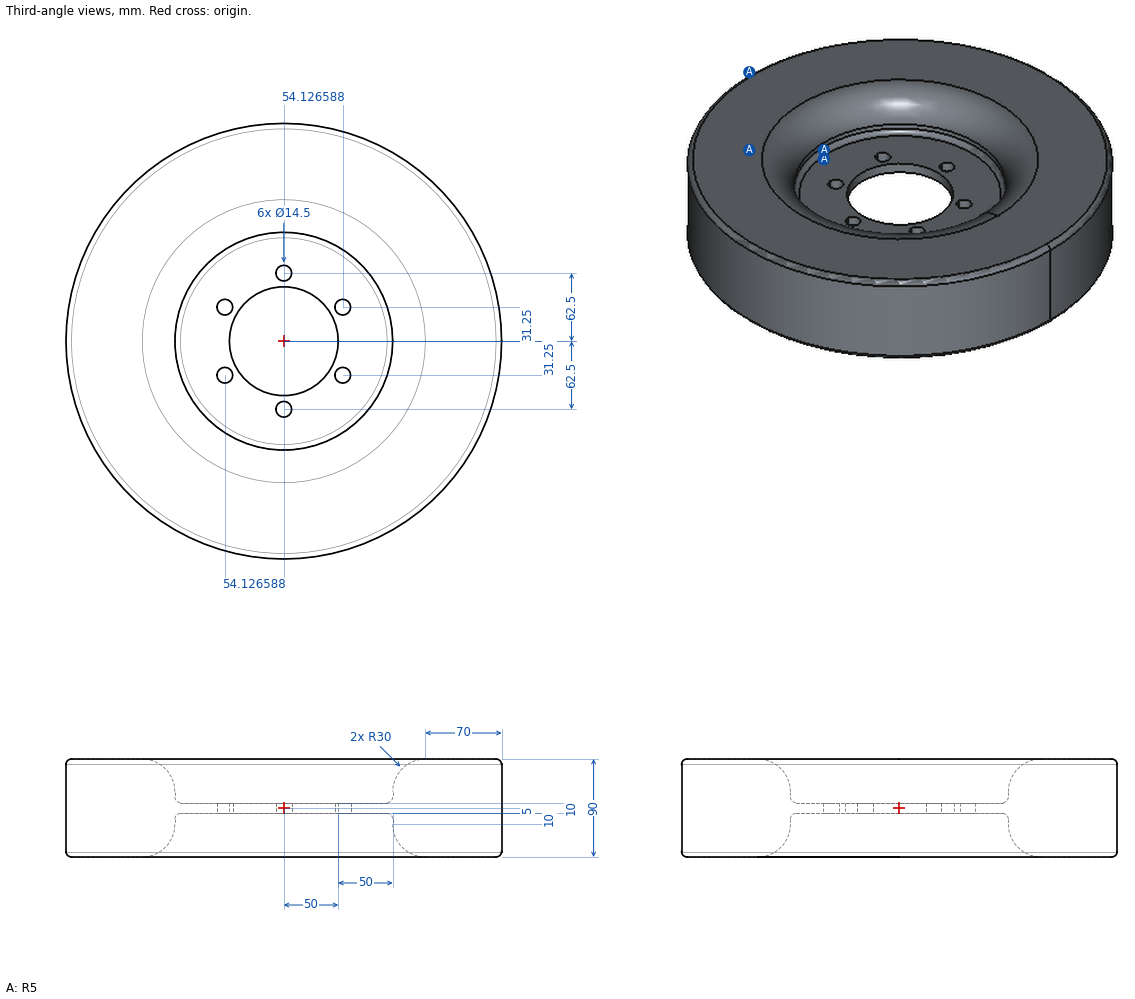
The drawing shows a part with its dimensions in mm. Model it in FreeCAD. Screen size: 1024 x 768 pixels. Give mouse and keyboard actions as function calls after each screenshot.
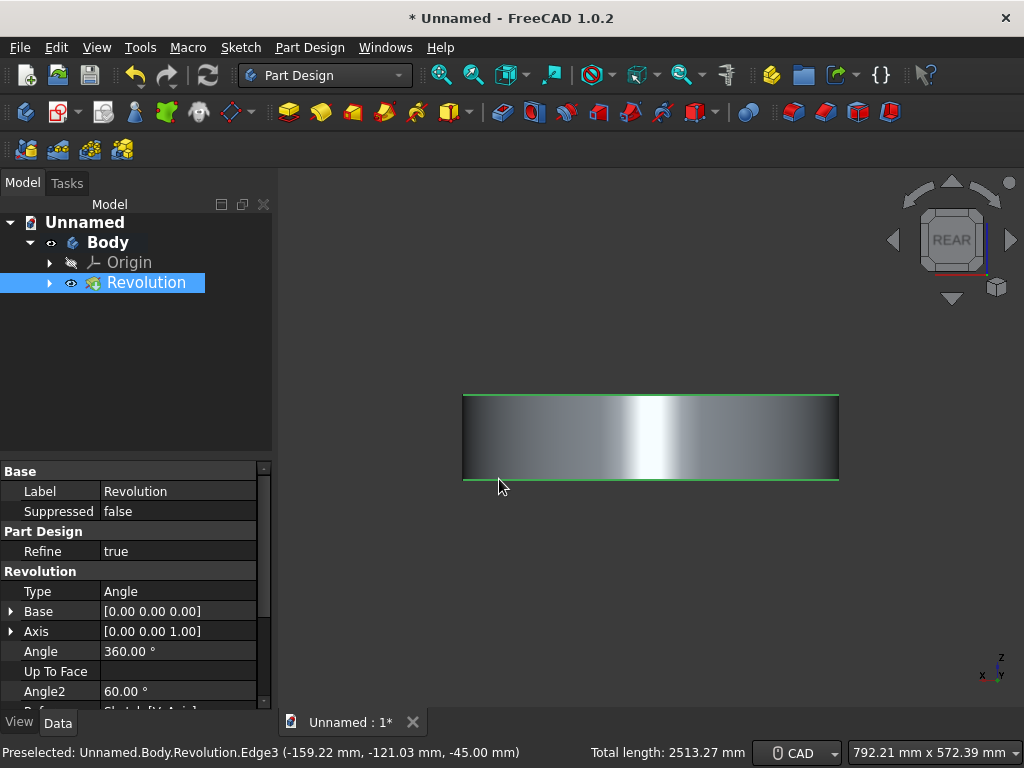
key(6)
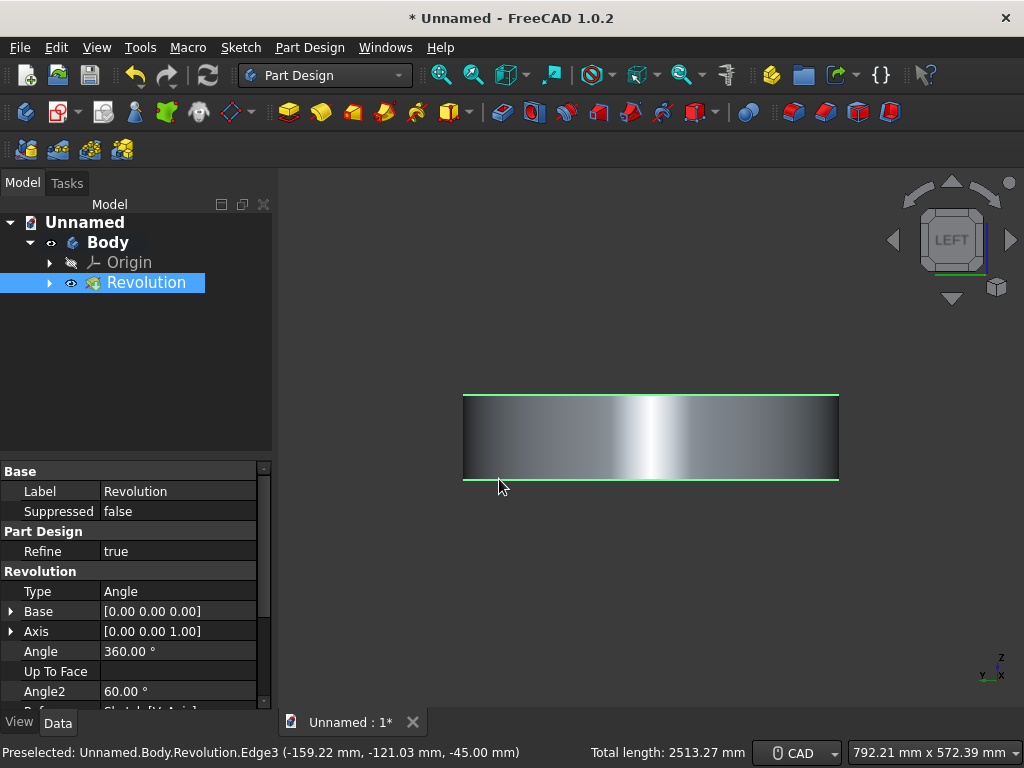
key(v)
key(3)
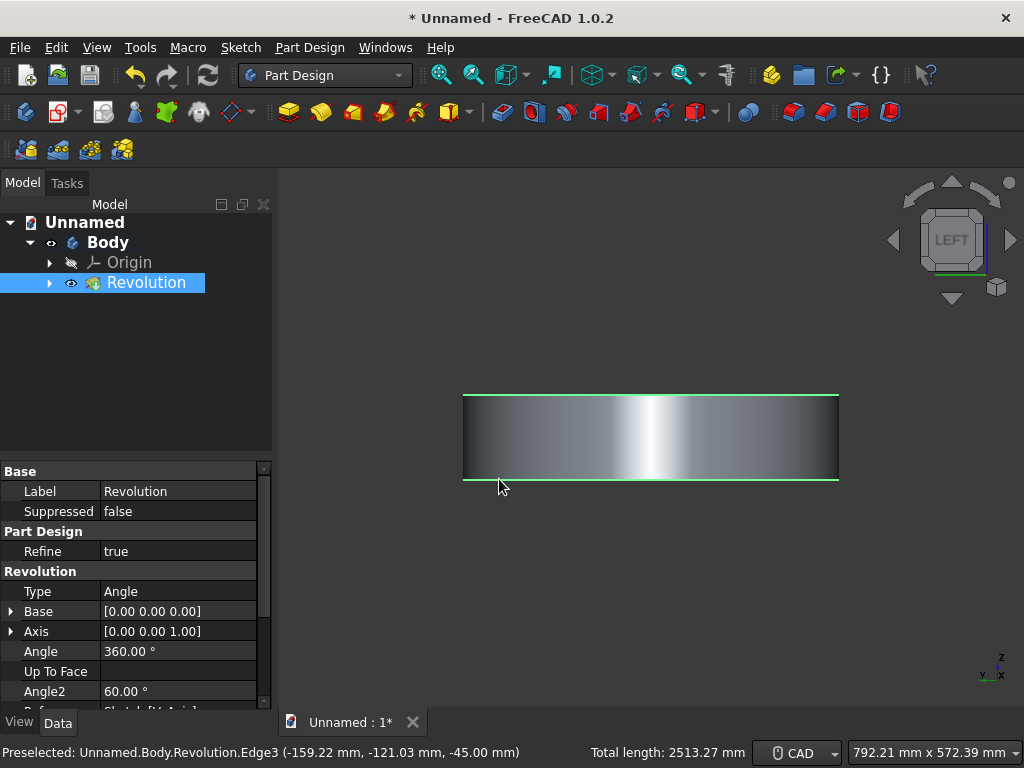
key(0)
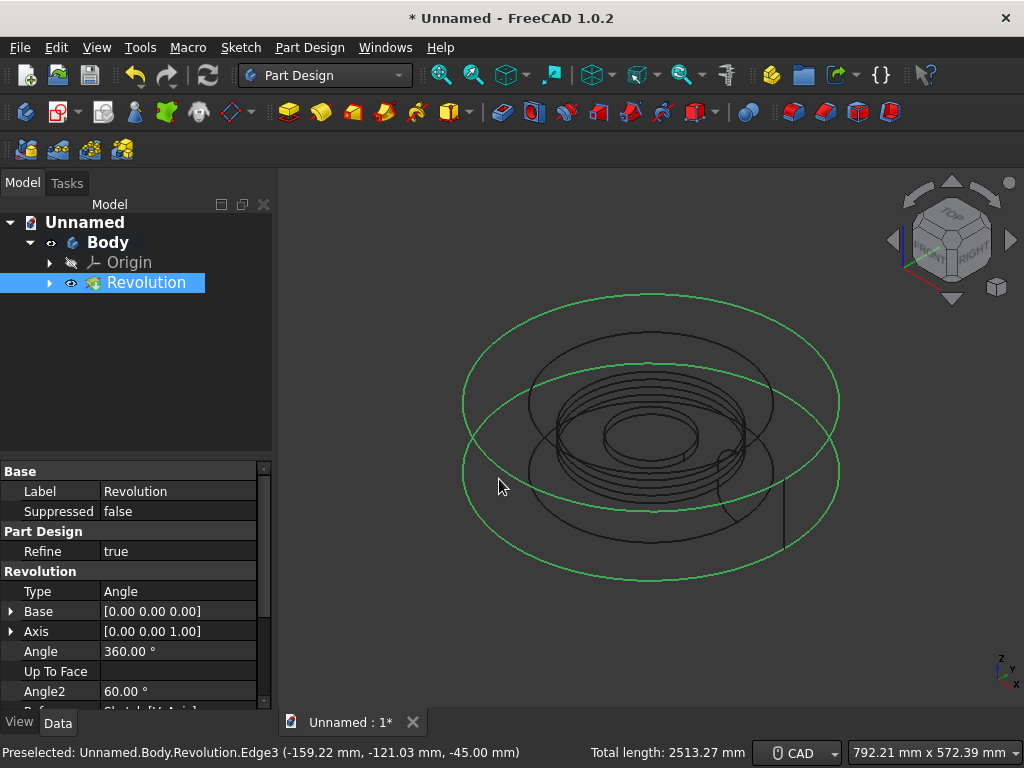
click(636, 387, ctrl)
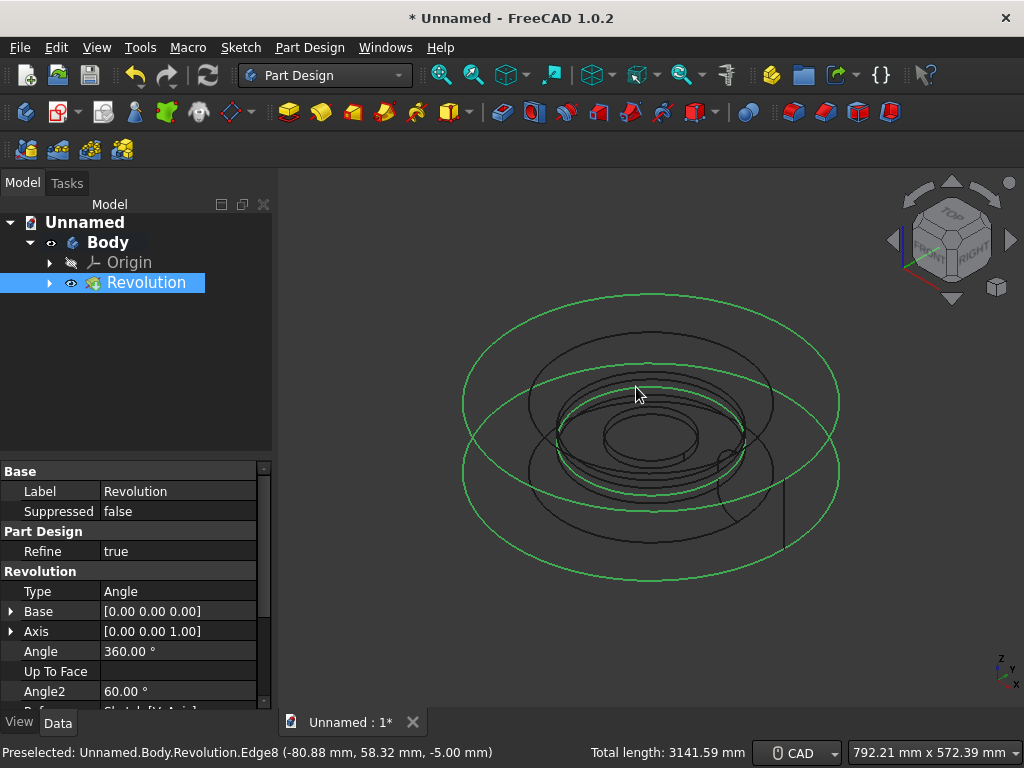
click(636, 379, ctrl)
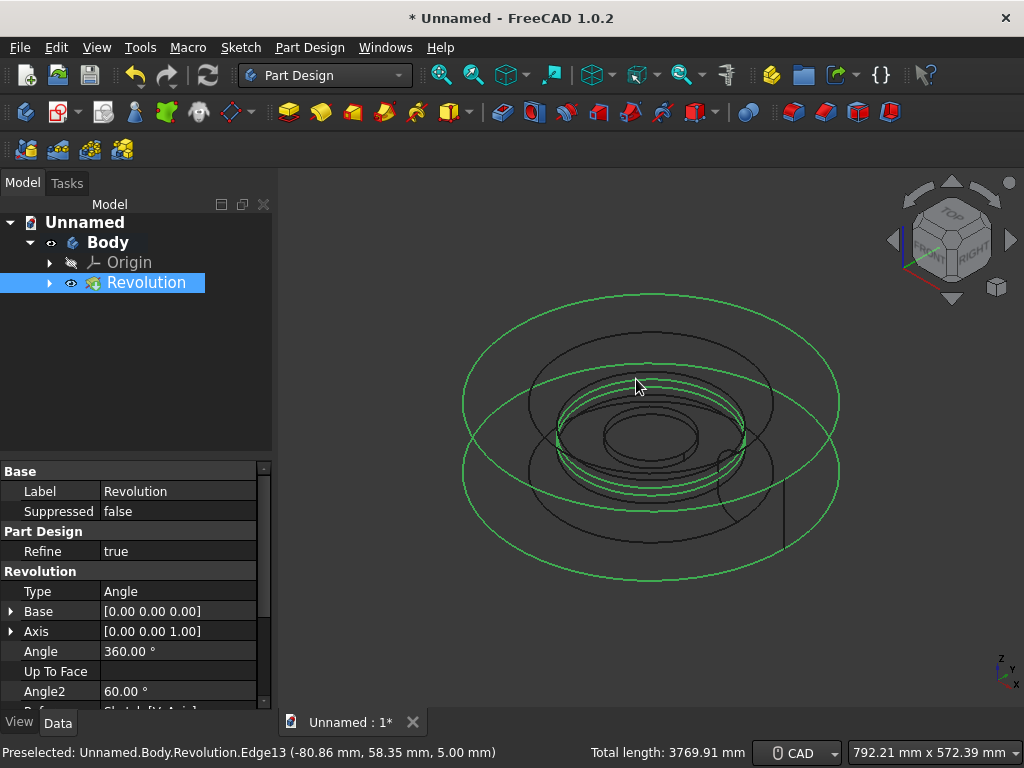
key(v)
key(1)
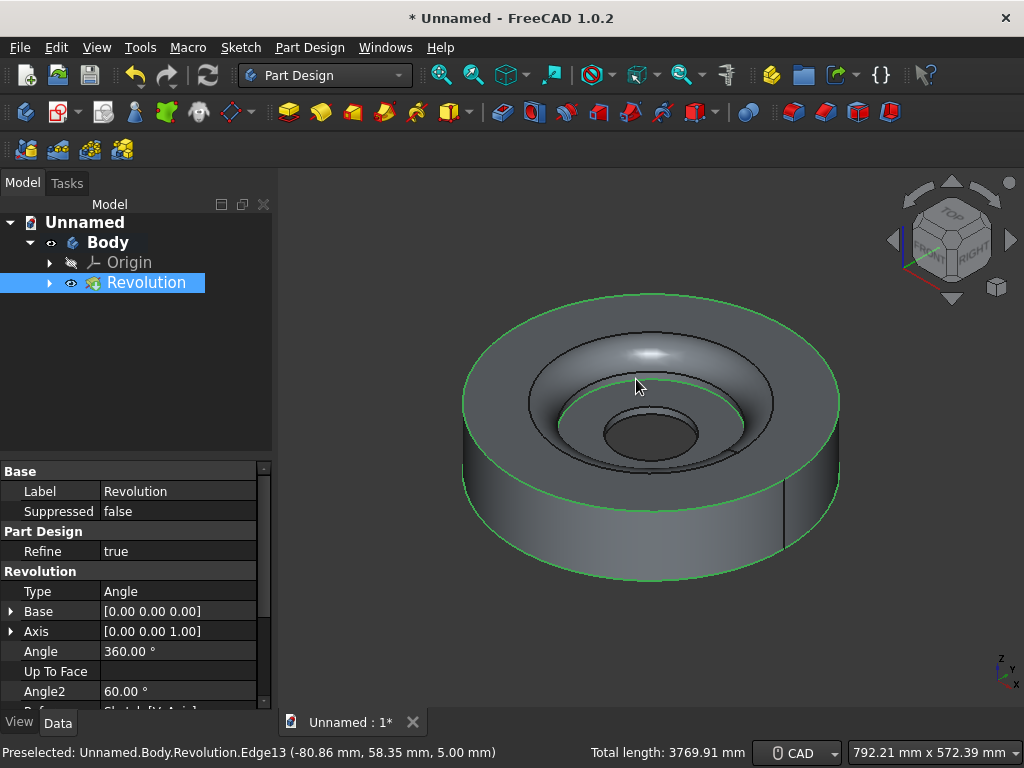
click(794, 112)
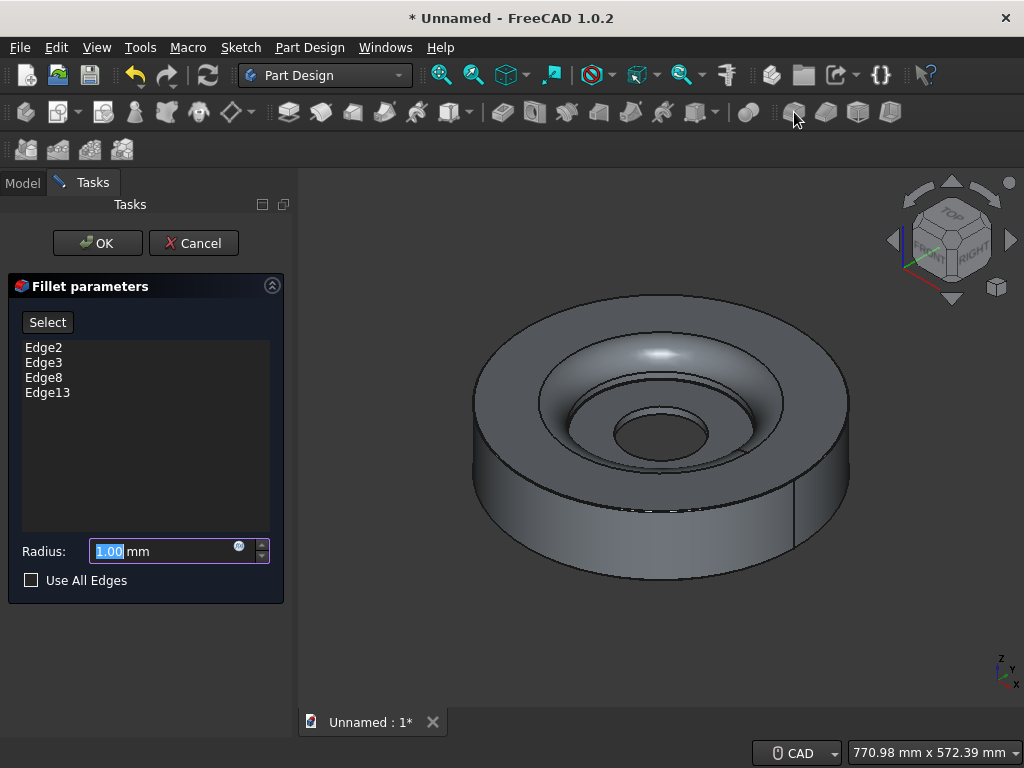
text(5)
key(Tab)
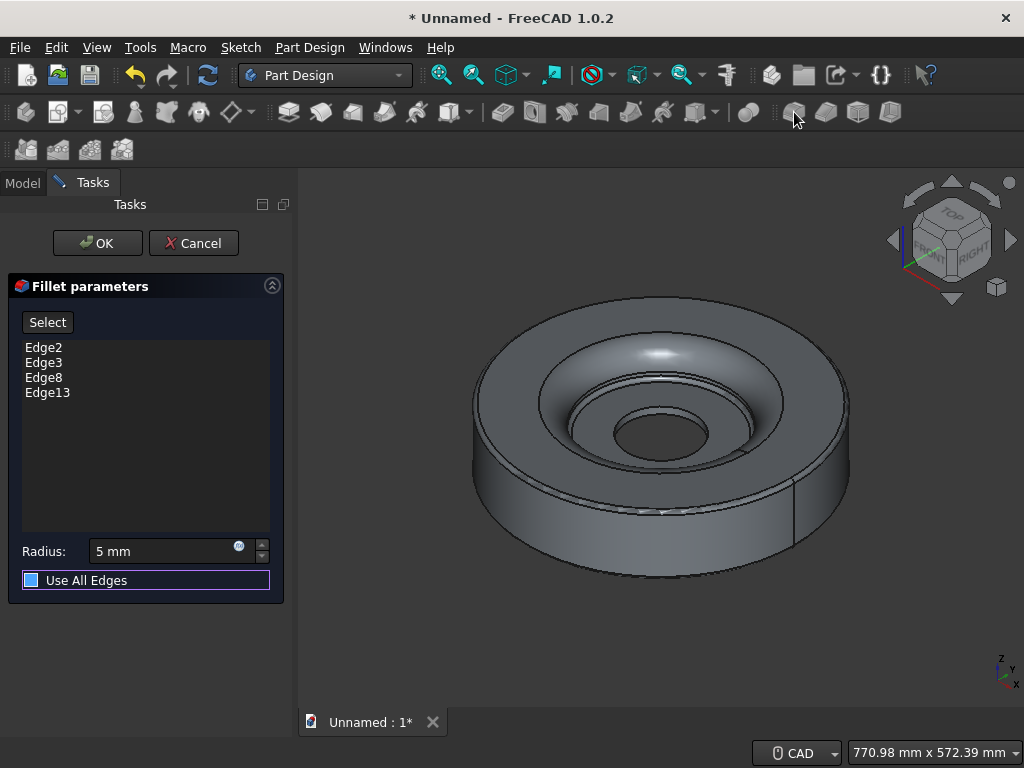
click(98, 243)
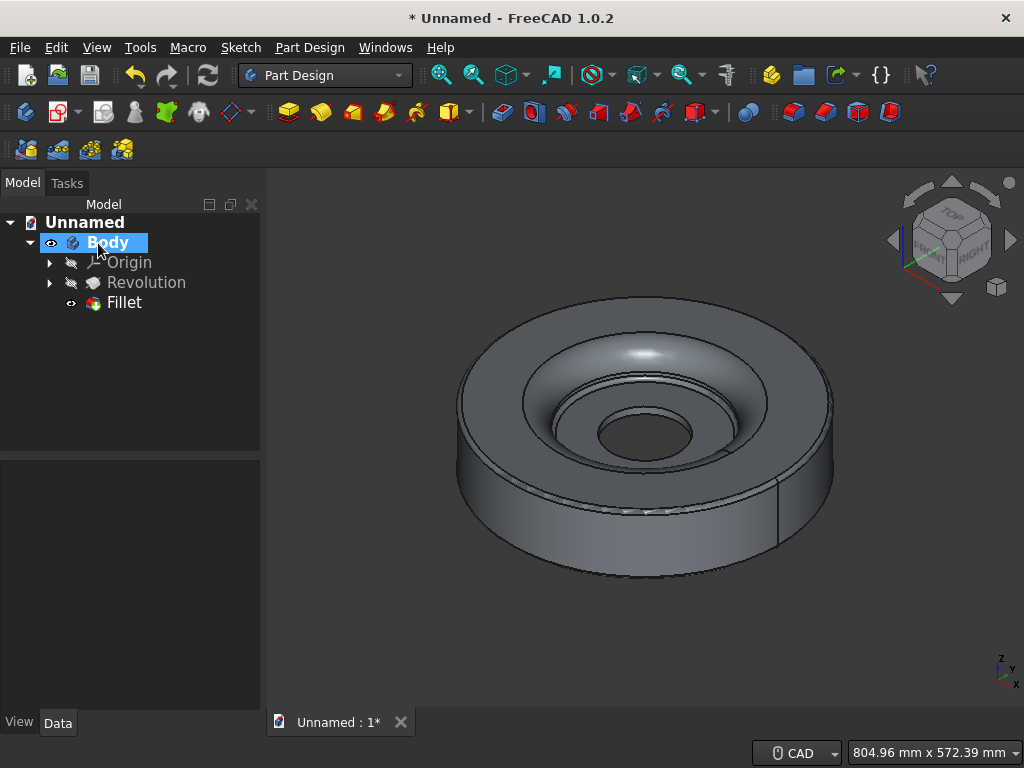
click(645, 391)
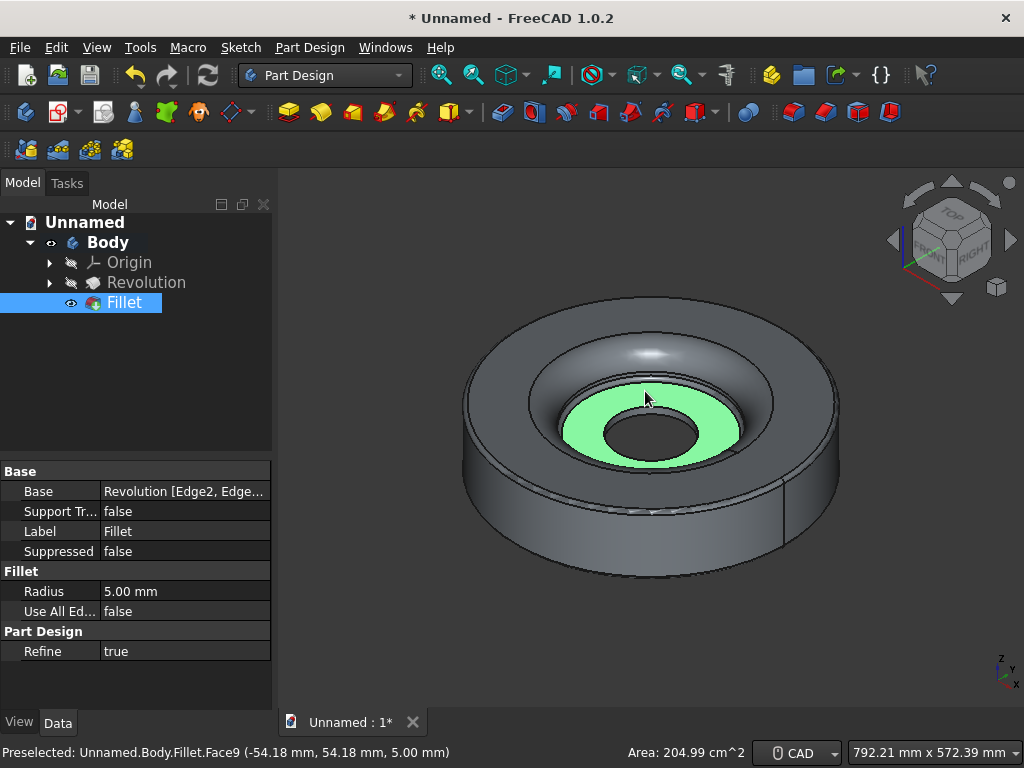
click(58, 112)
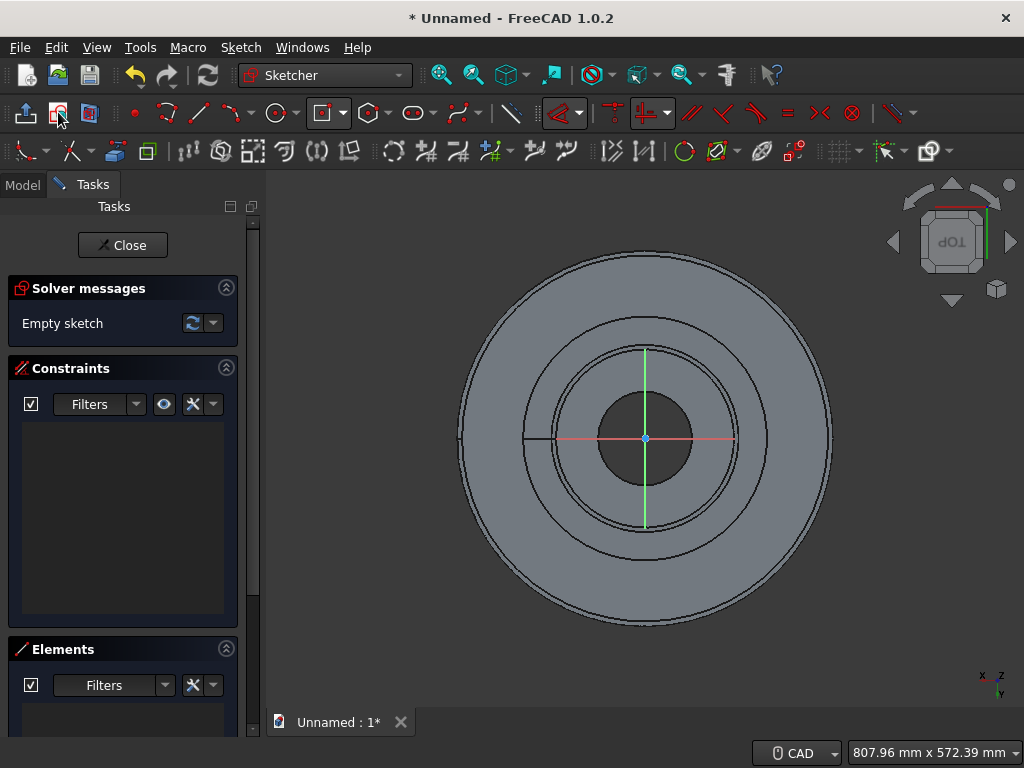
scroll(685, 439, up, 5)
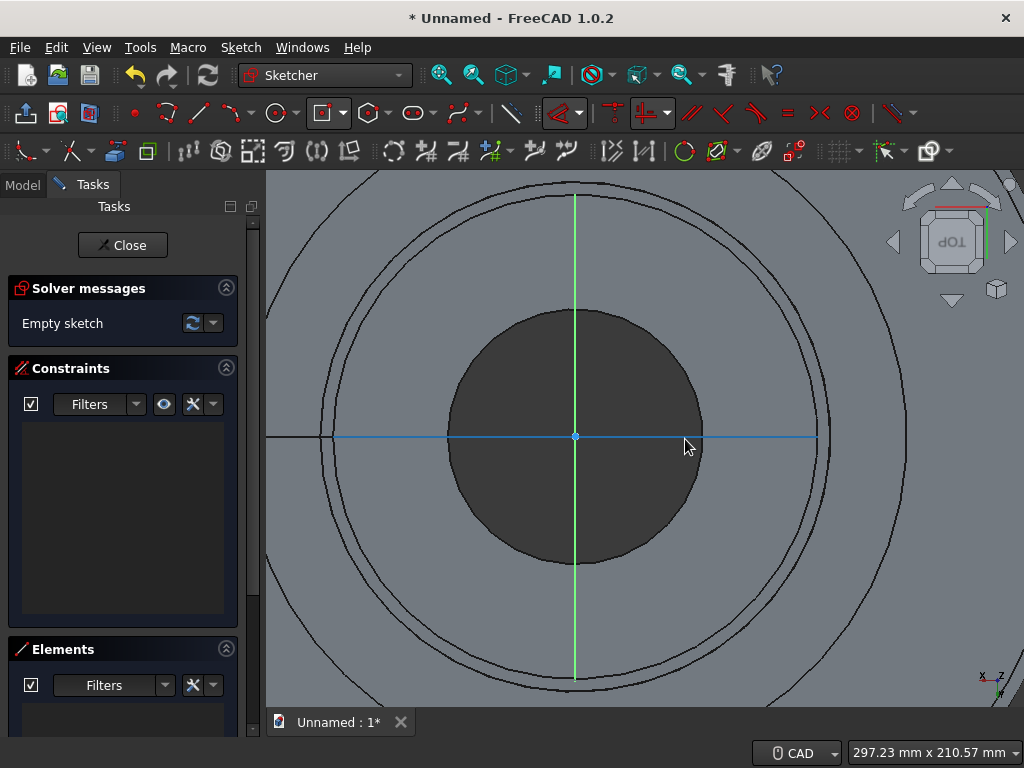
click(276, 114)